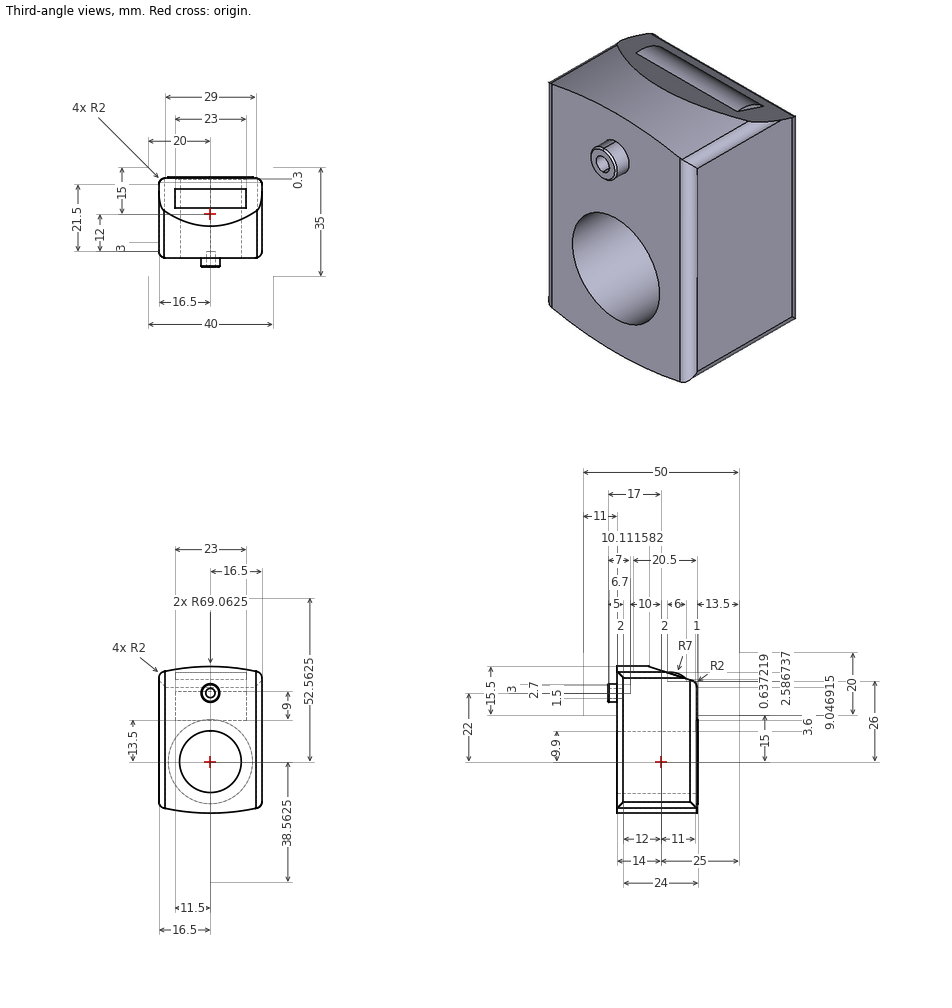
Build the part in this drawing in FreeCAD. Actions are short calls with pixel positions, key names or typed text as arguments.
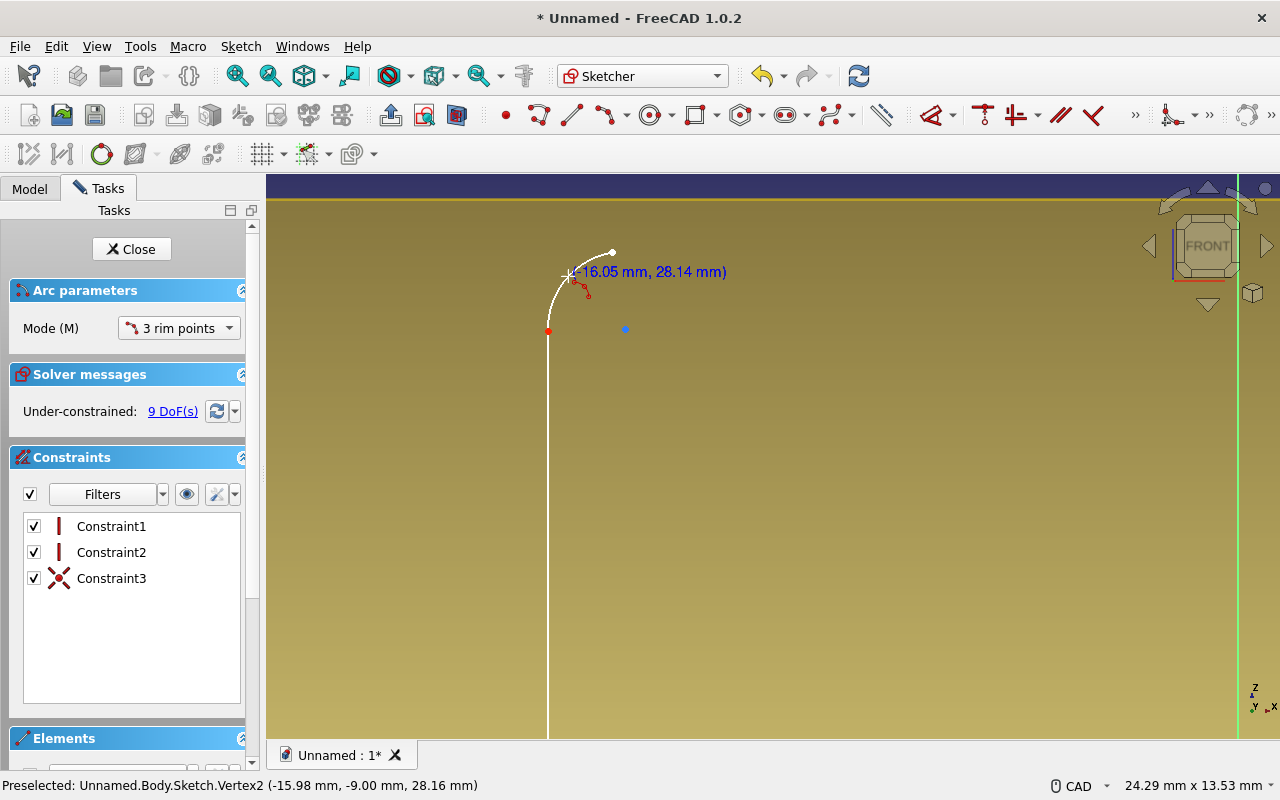
scroll(570, 279, down, 8)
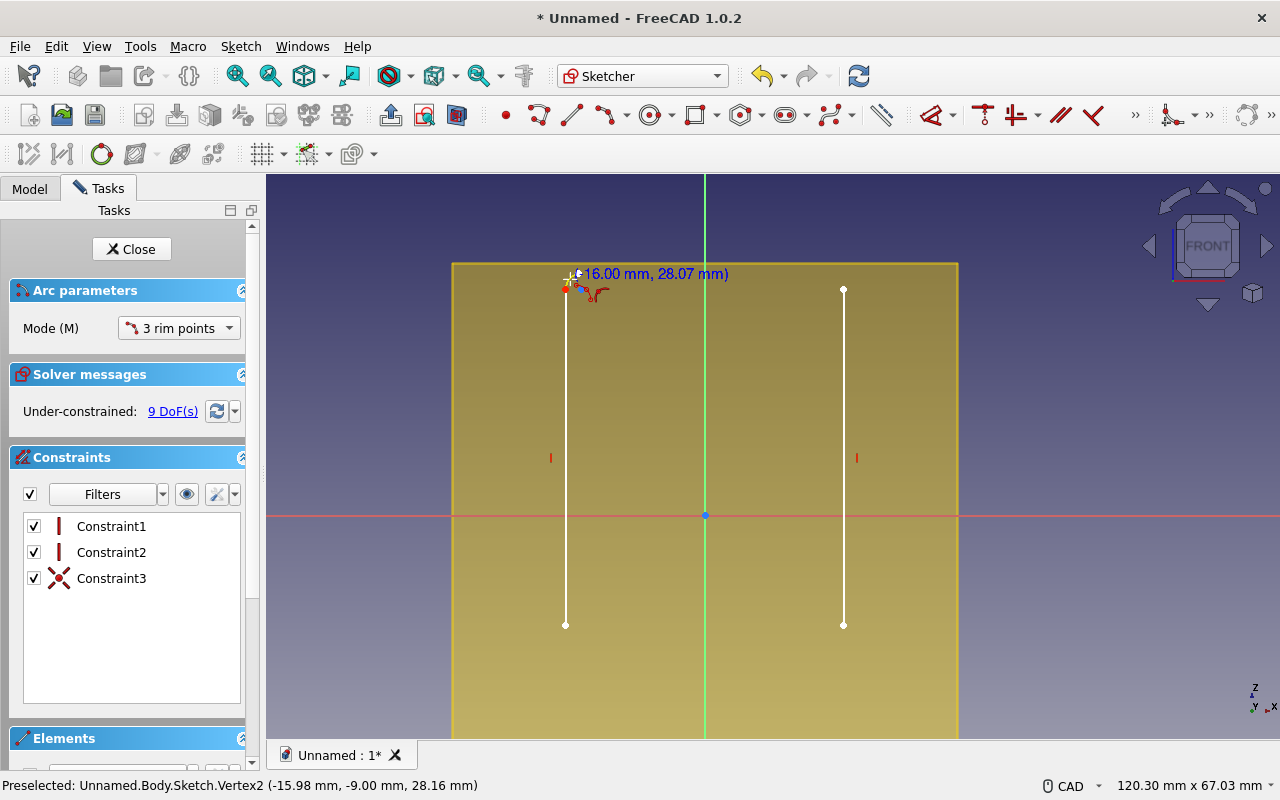
click(579, 274)
click(831, 273)
click(730, 259)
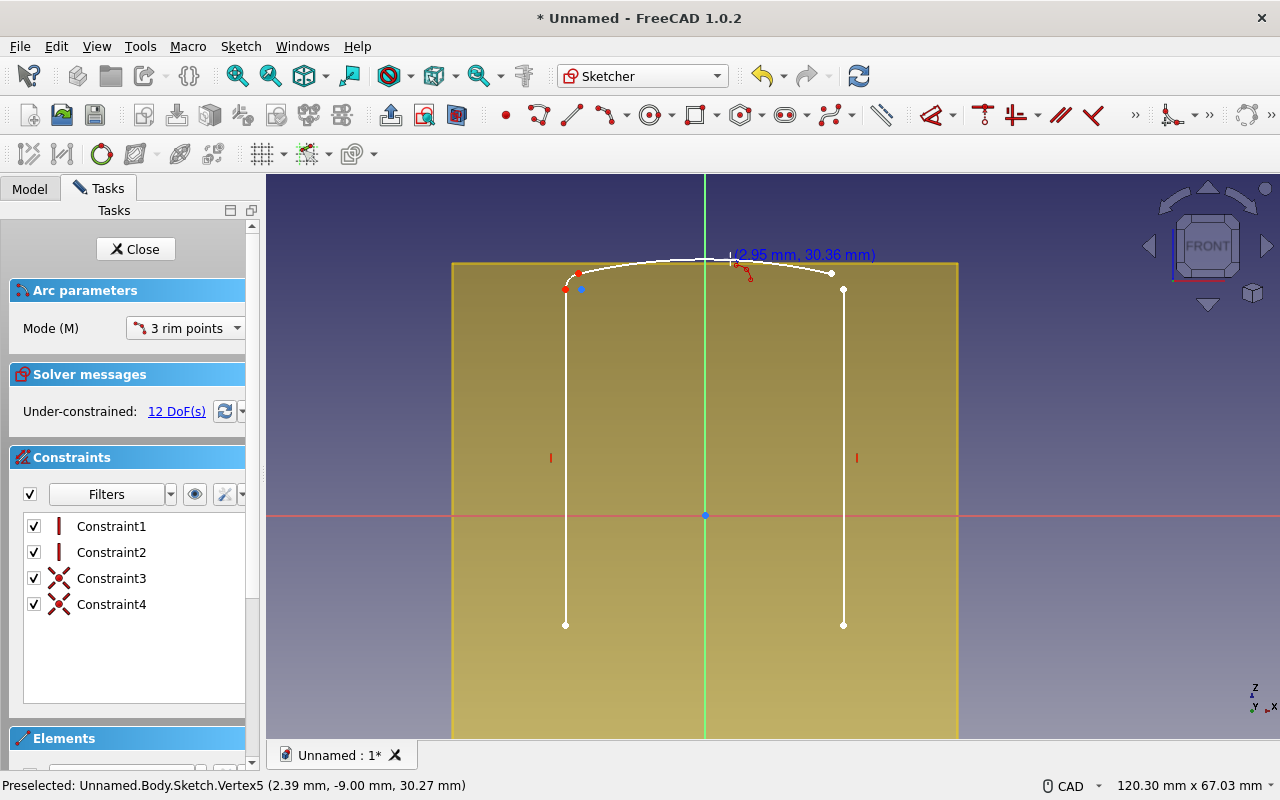
click(831, 274)
click(844, 290)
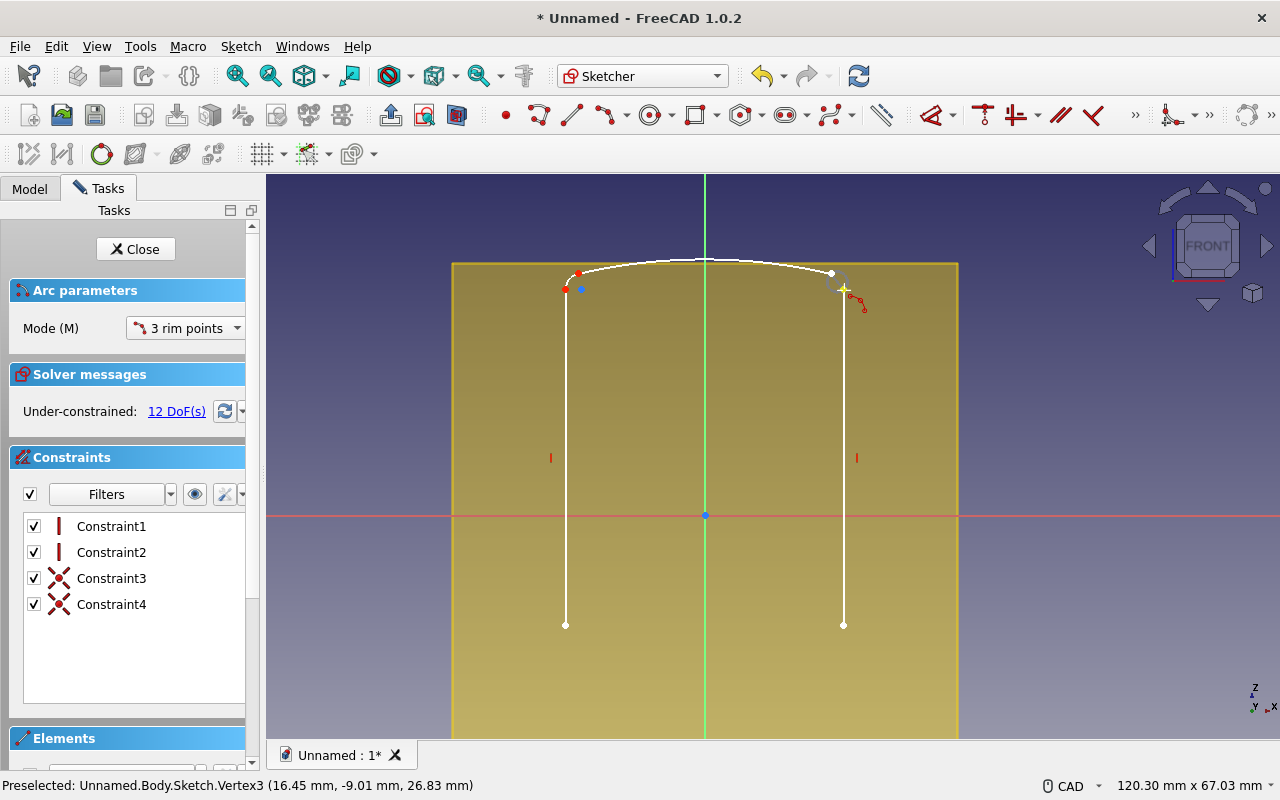
scroll(840, 279, up, 8)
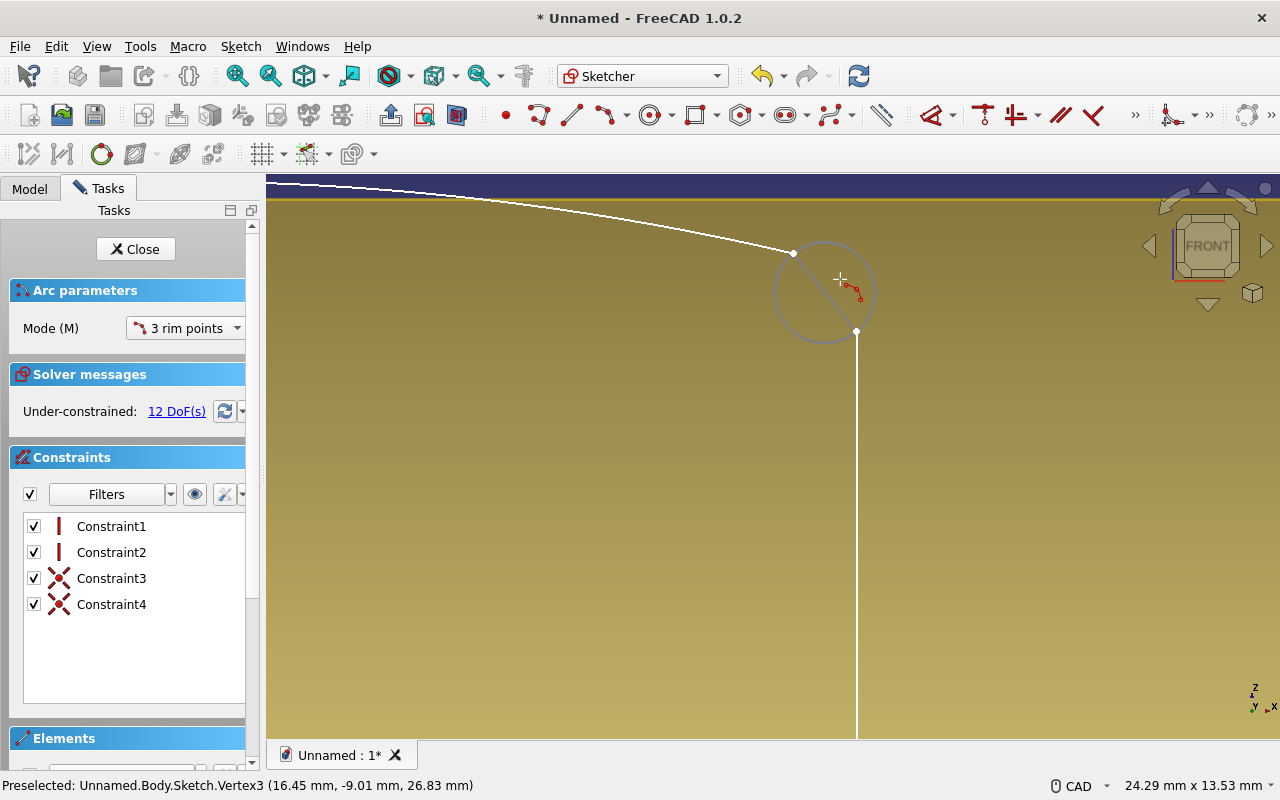
click(840, 276)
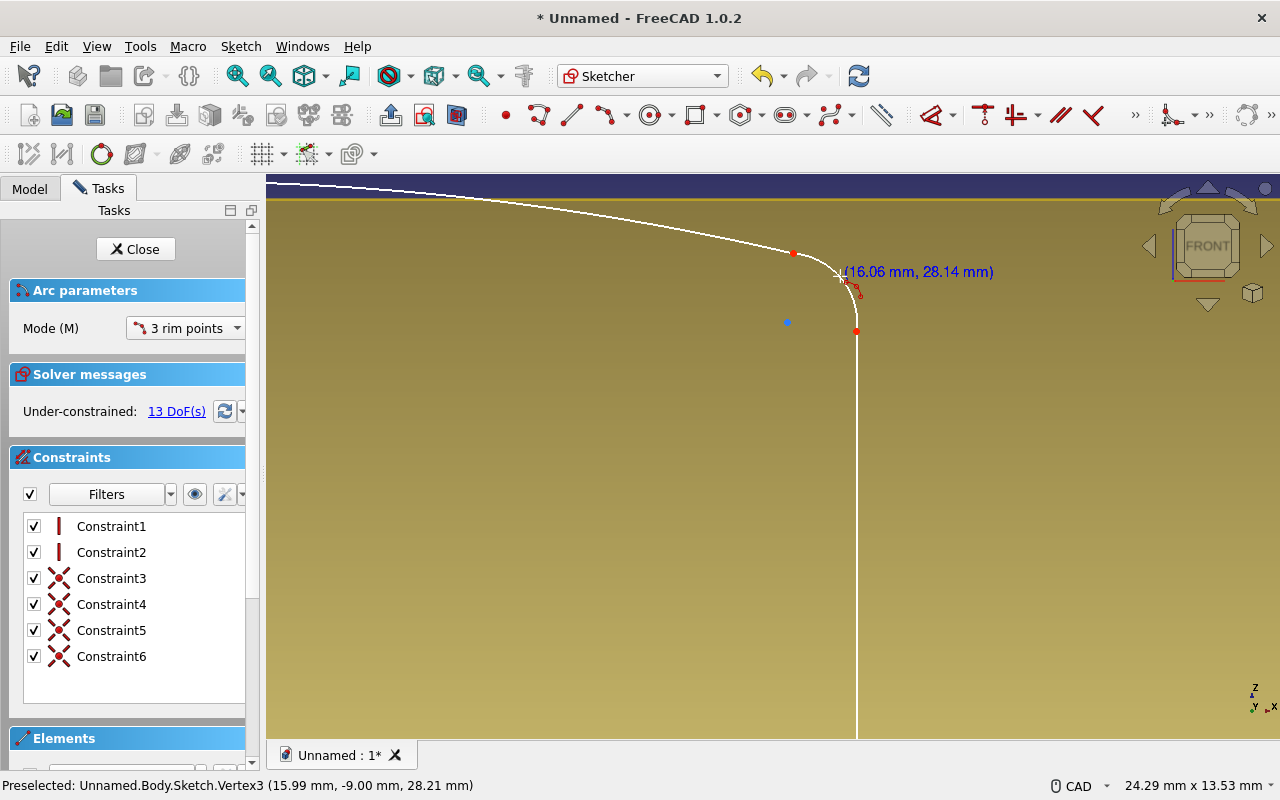
scroll(840, 279, down, 8)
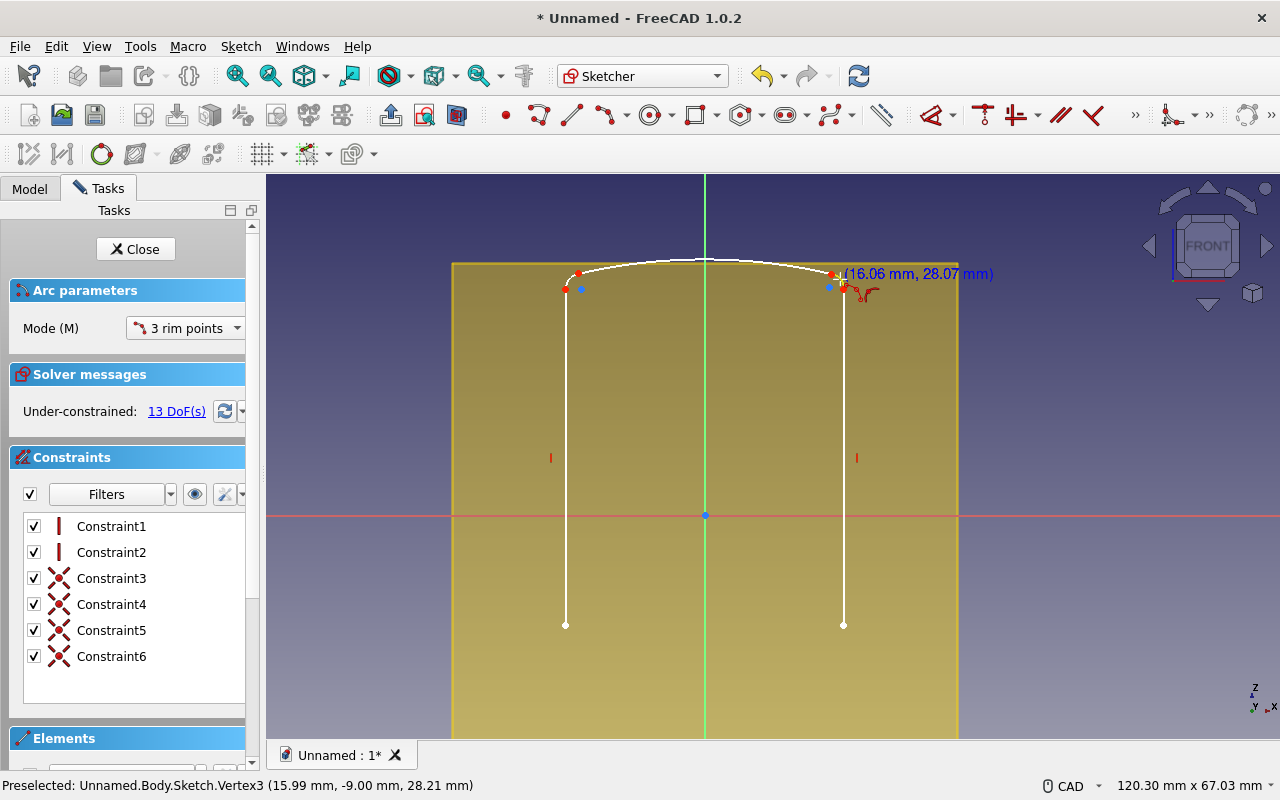
click(844, 626)
click(831, 641)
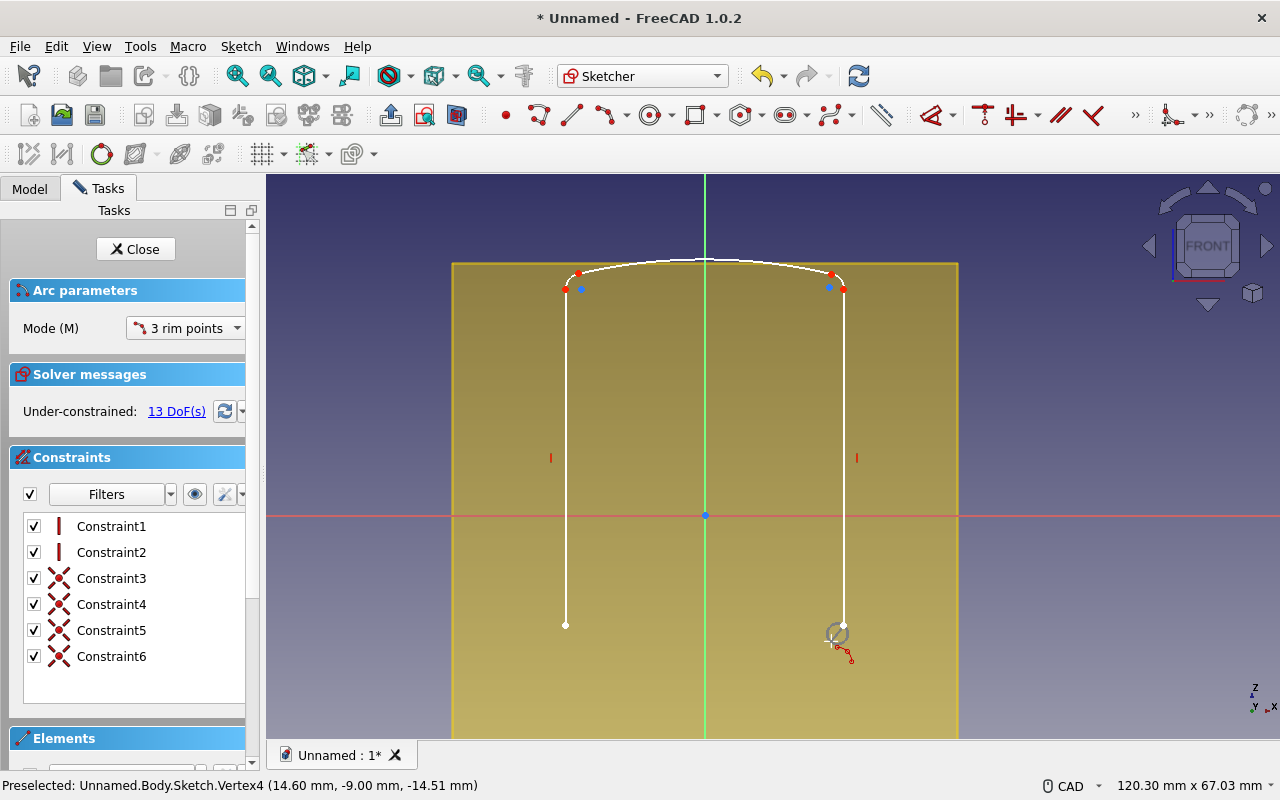
scroll(840, 635, up, 8)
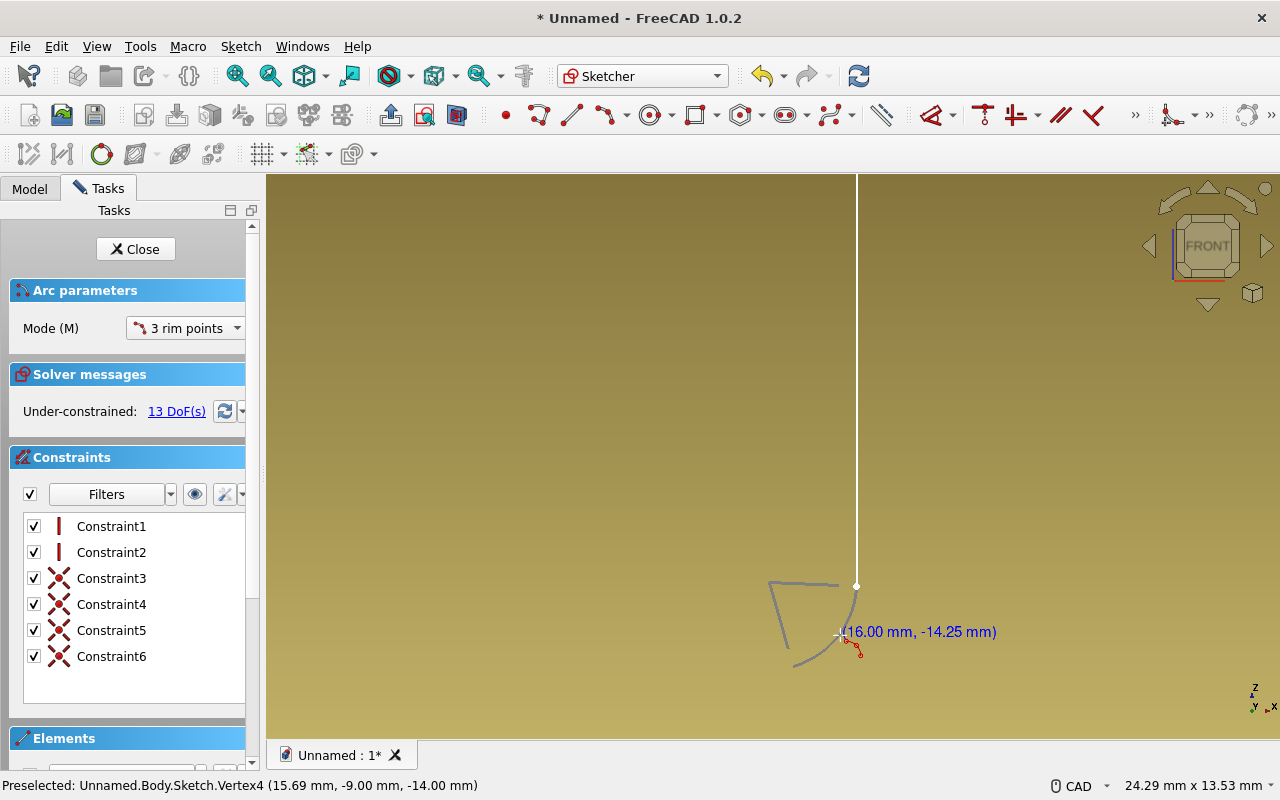
click(840, 633)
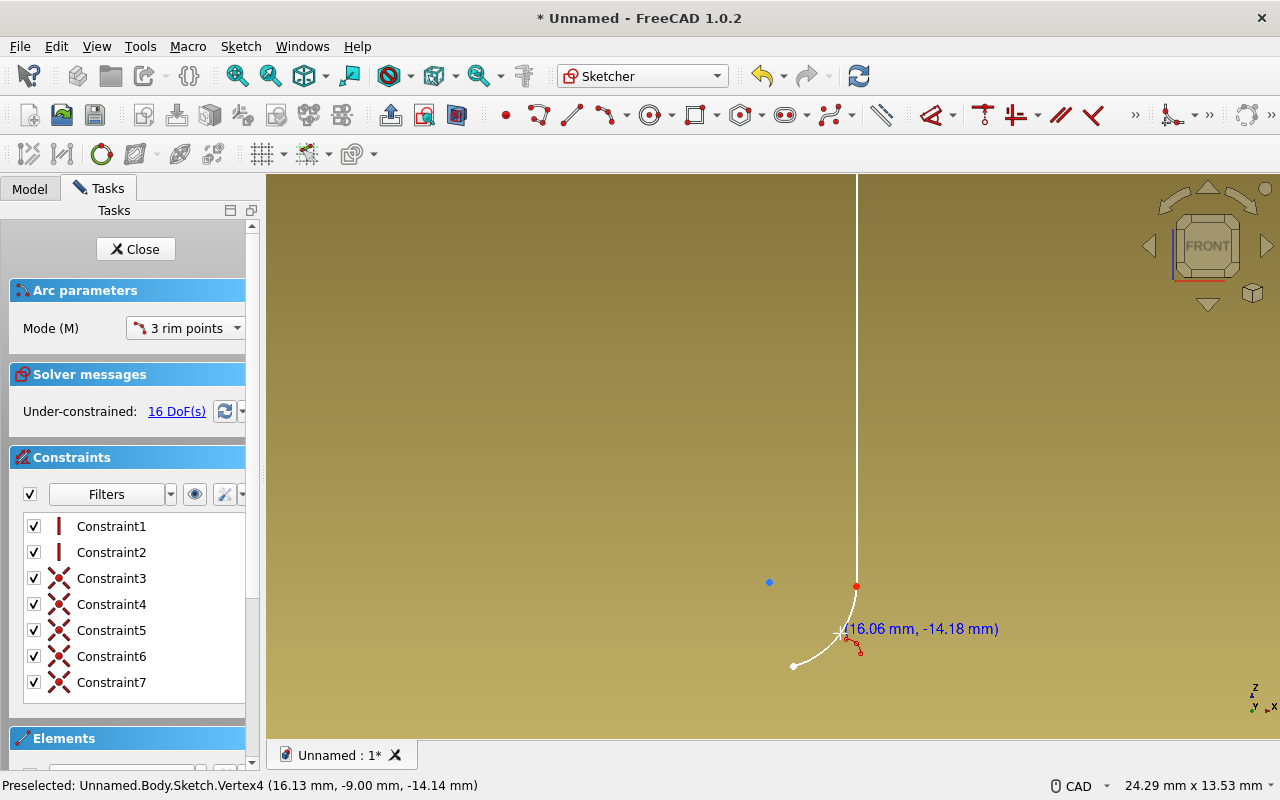
scroll(840, 635, down, 8)